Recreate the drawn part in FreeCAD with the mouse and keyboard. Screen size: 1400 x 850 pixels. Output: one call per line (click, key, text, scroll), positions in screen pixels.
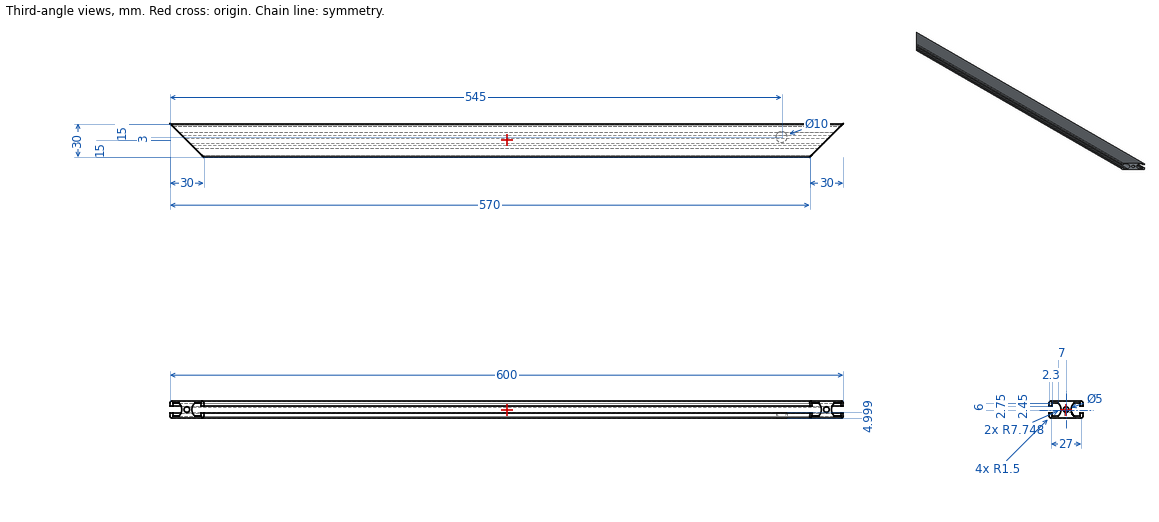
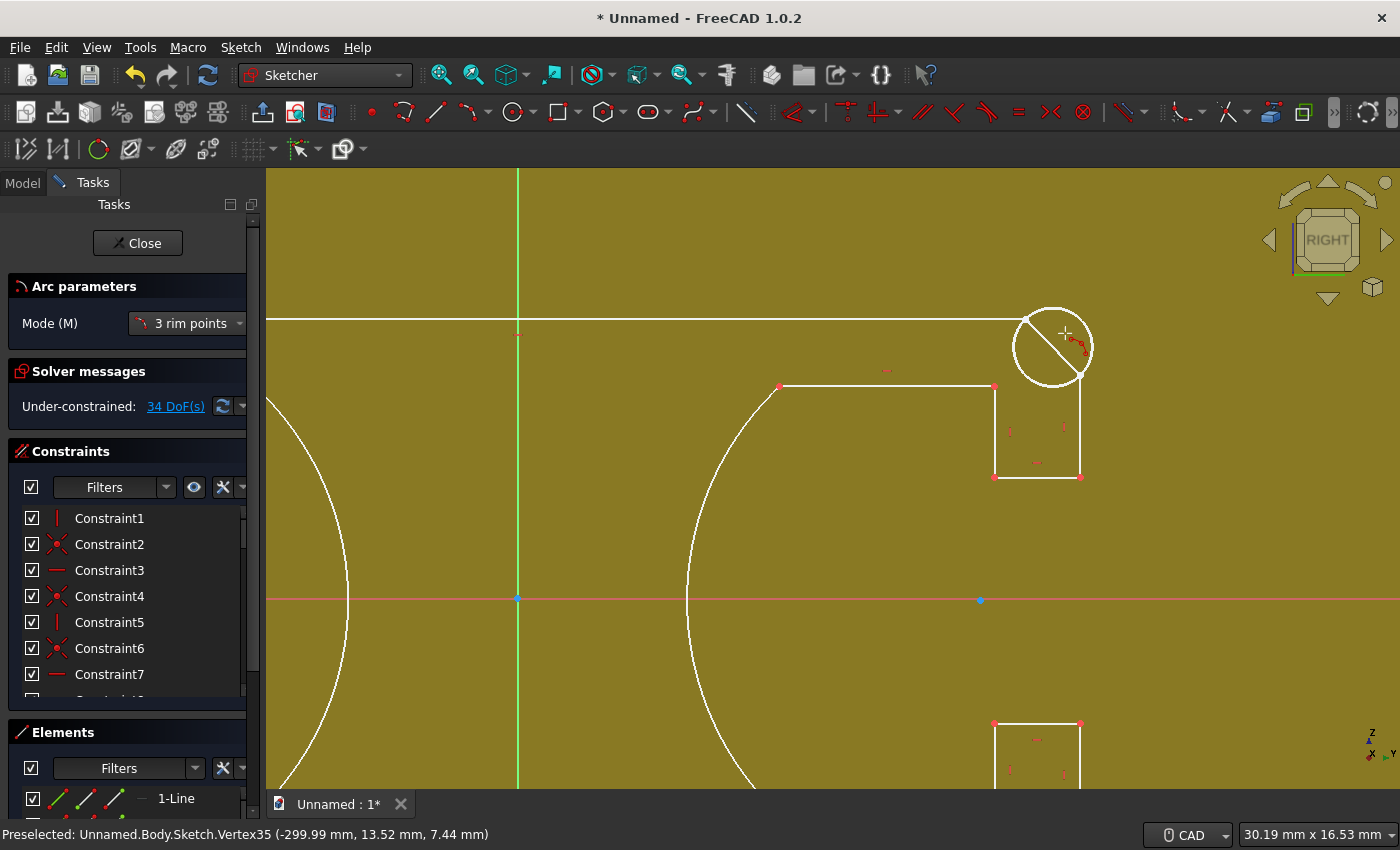
click(1065, 333)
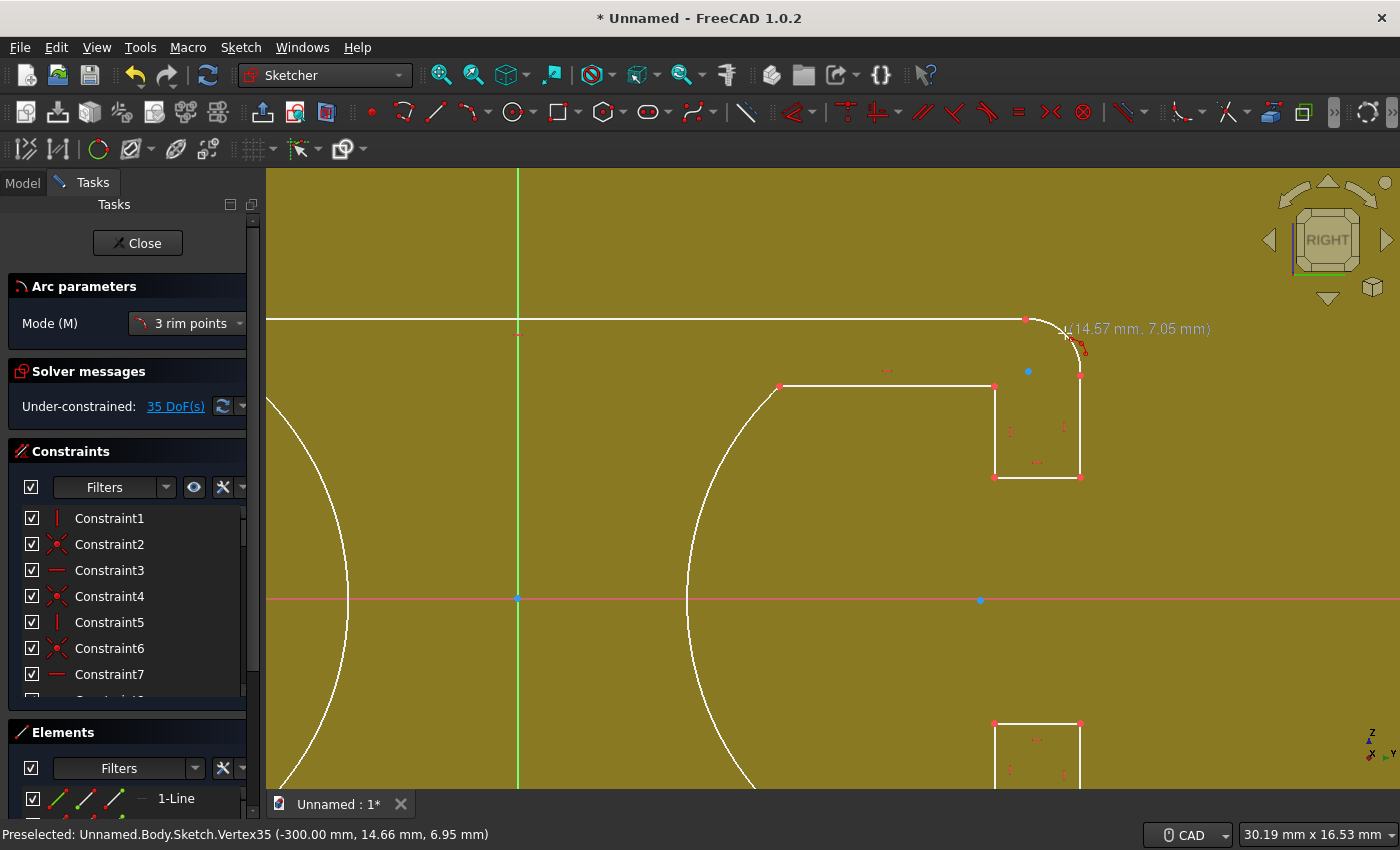
scroll(1065, 332, down, 3)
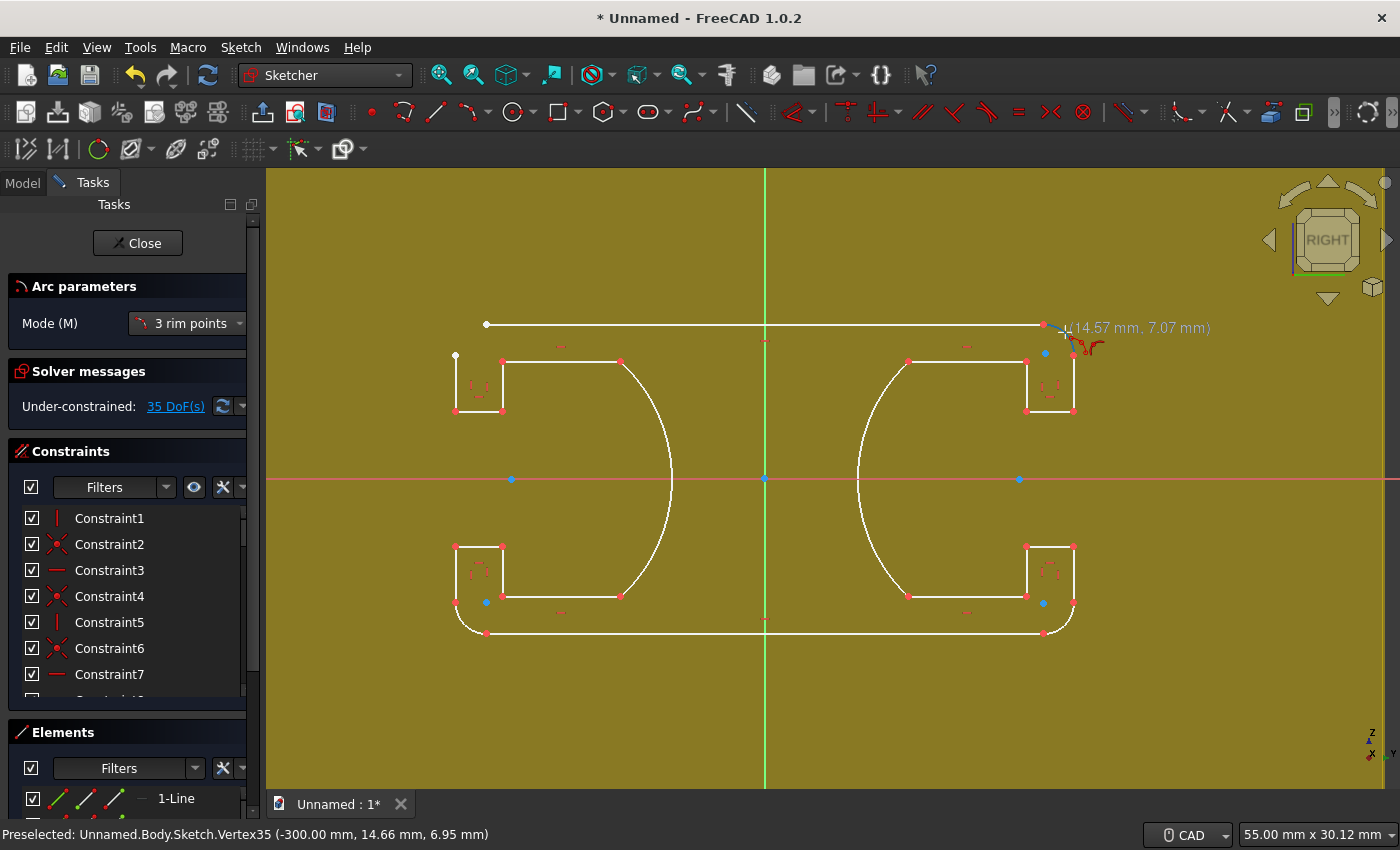
click(487, 325)
click(456, 356)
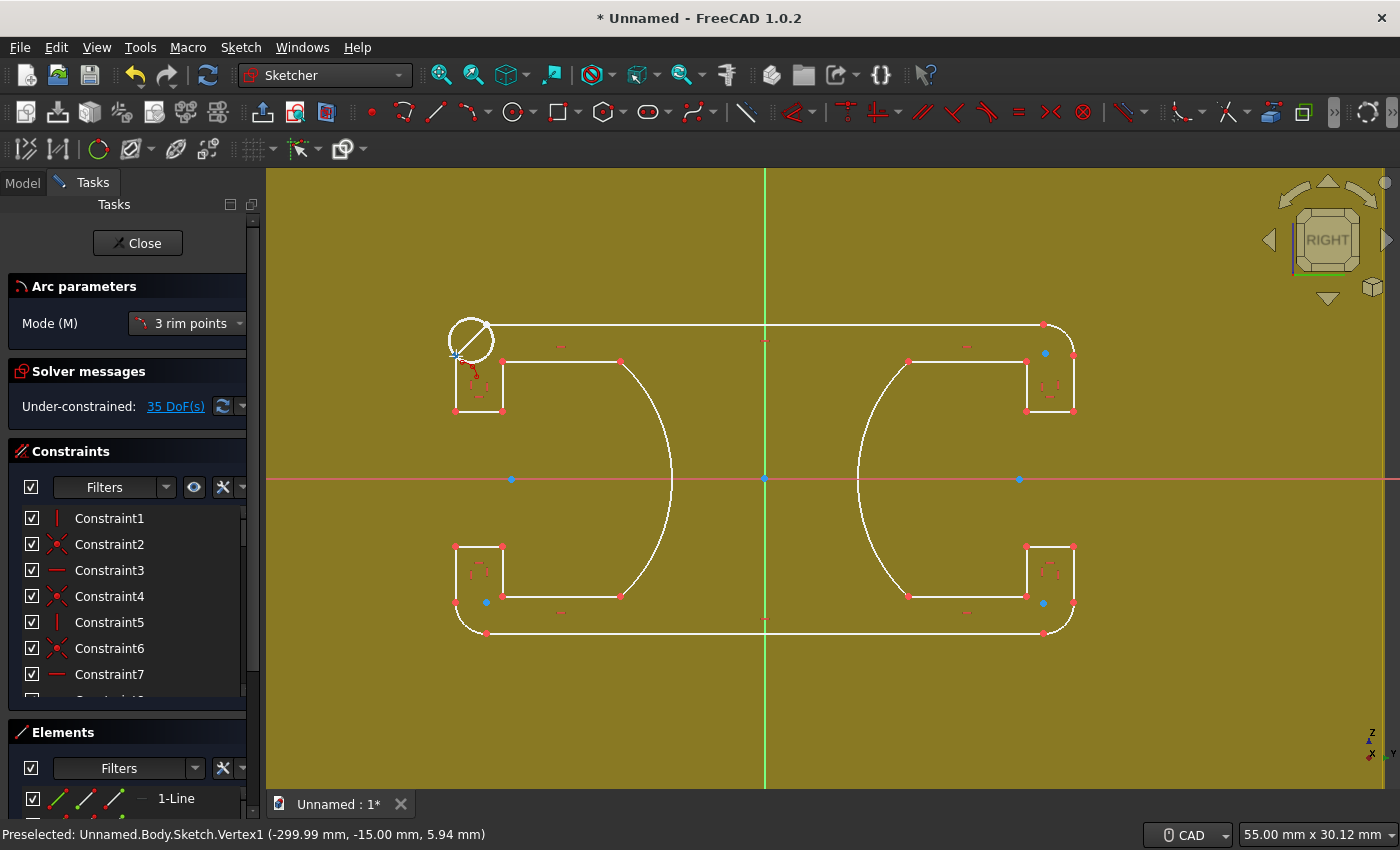
scroll(465, 333, up, 3)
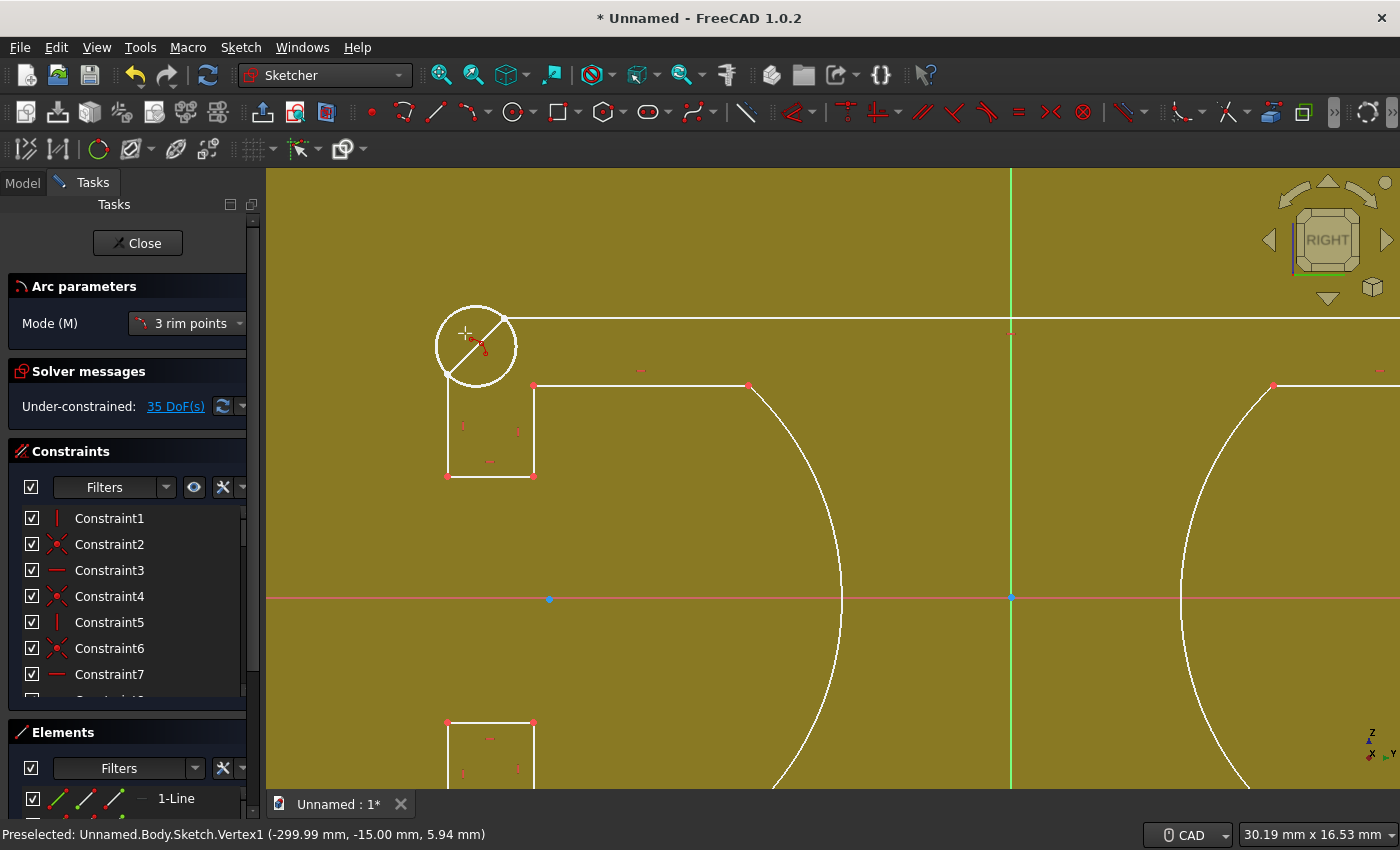
click(464, 333)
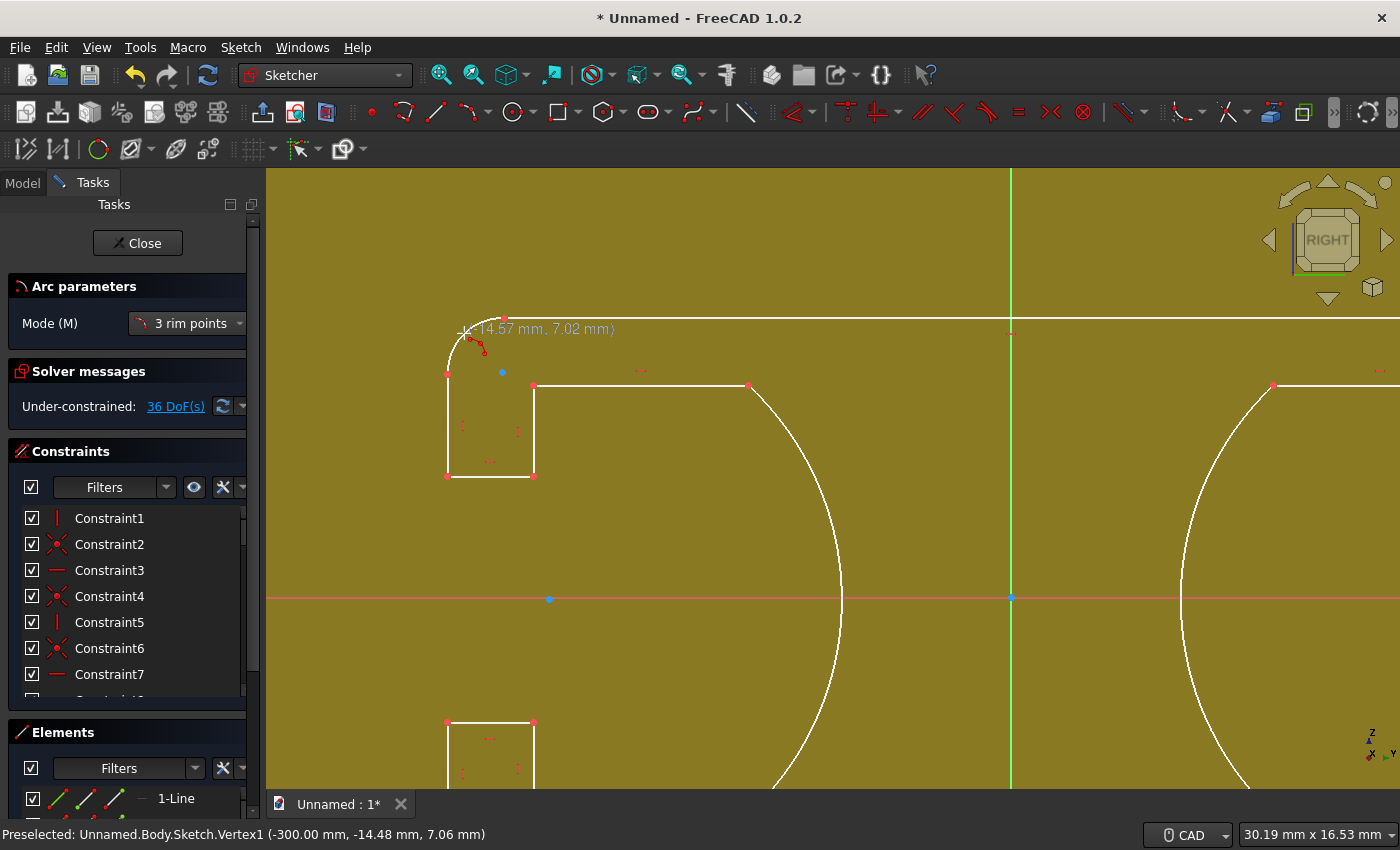
key(g)
key(c)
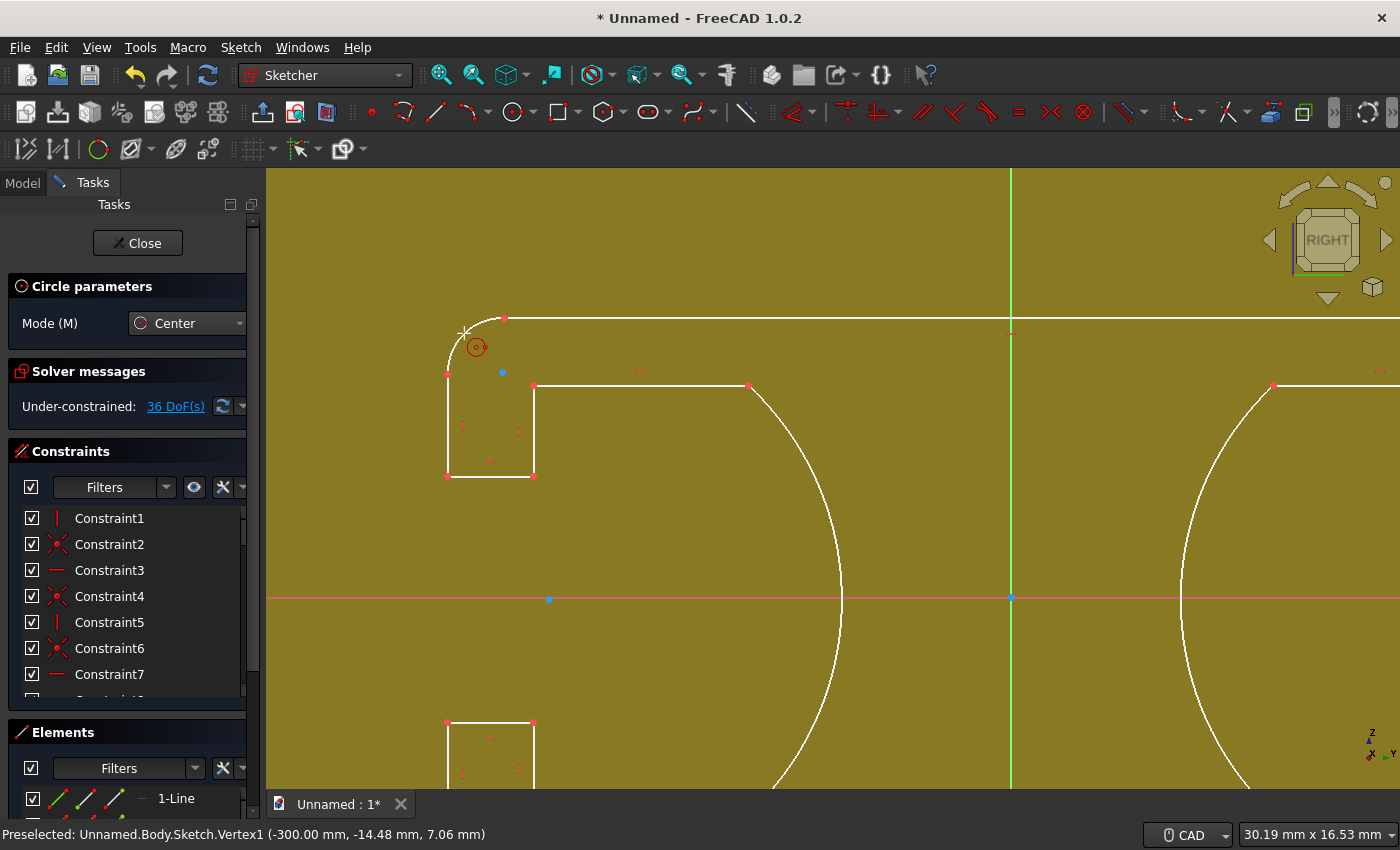
click(1011, 598)
move(1078, 531)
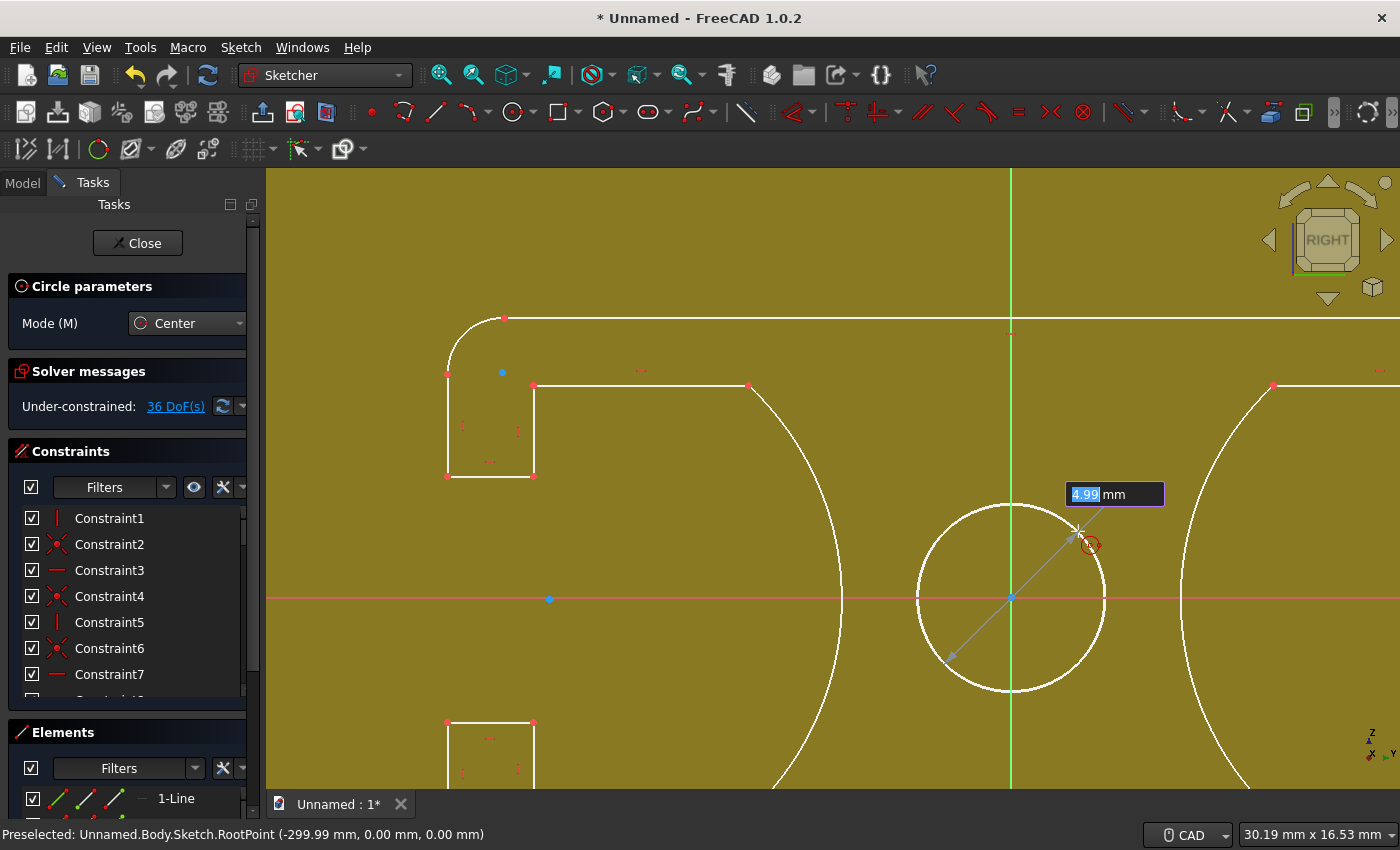
text(5)
key(Return)
key(Escape)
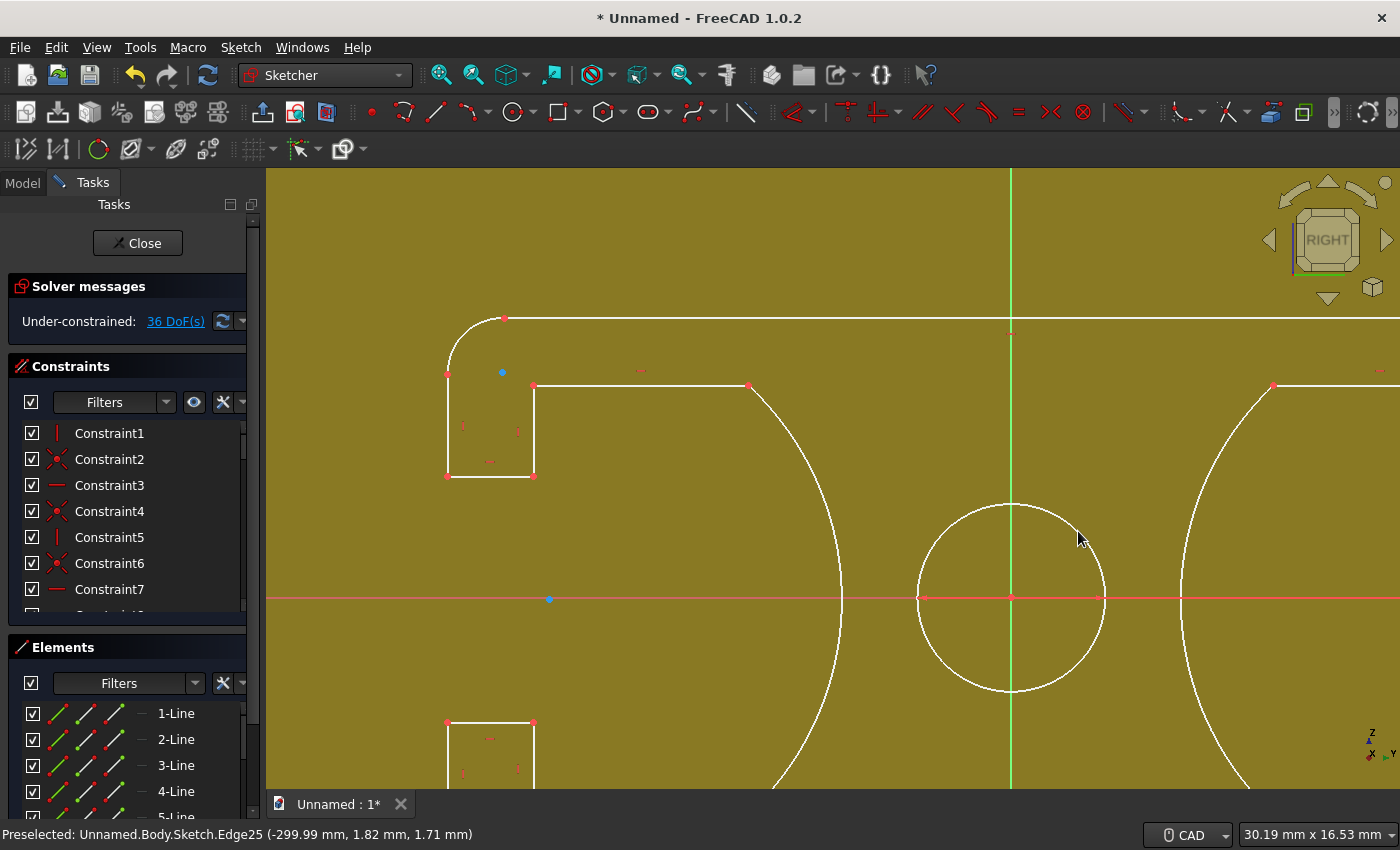
click(448, 405)